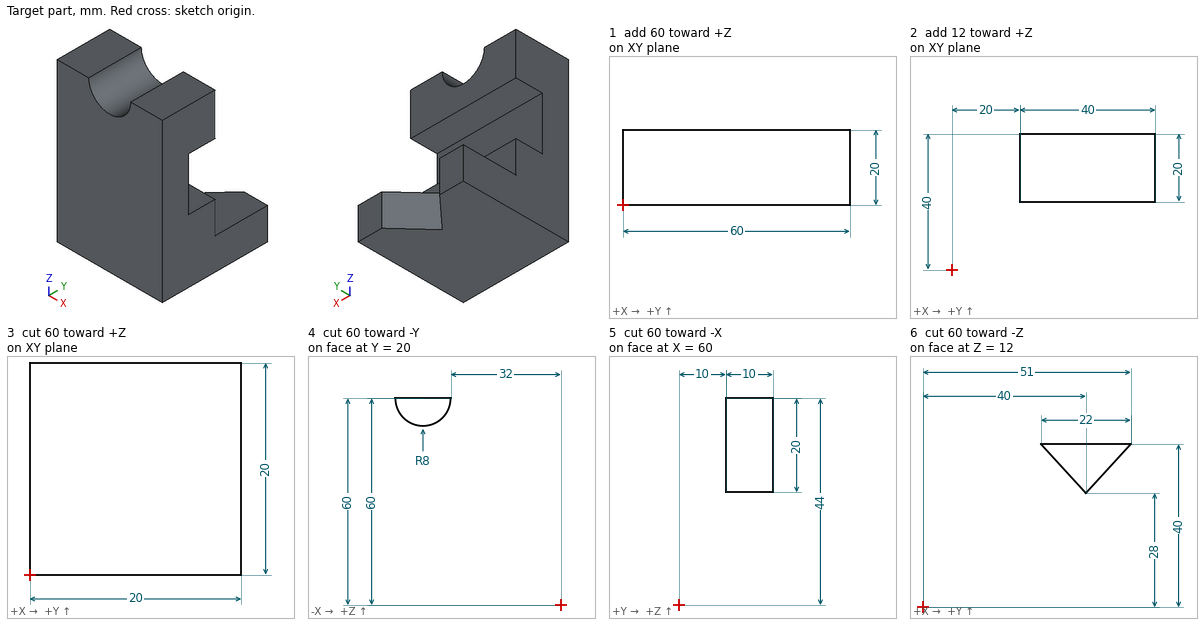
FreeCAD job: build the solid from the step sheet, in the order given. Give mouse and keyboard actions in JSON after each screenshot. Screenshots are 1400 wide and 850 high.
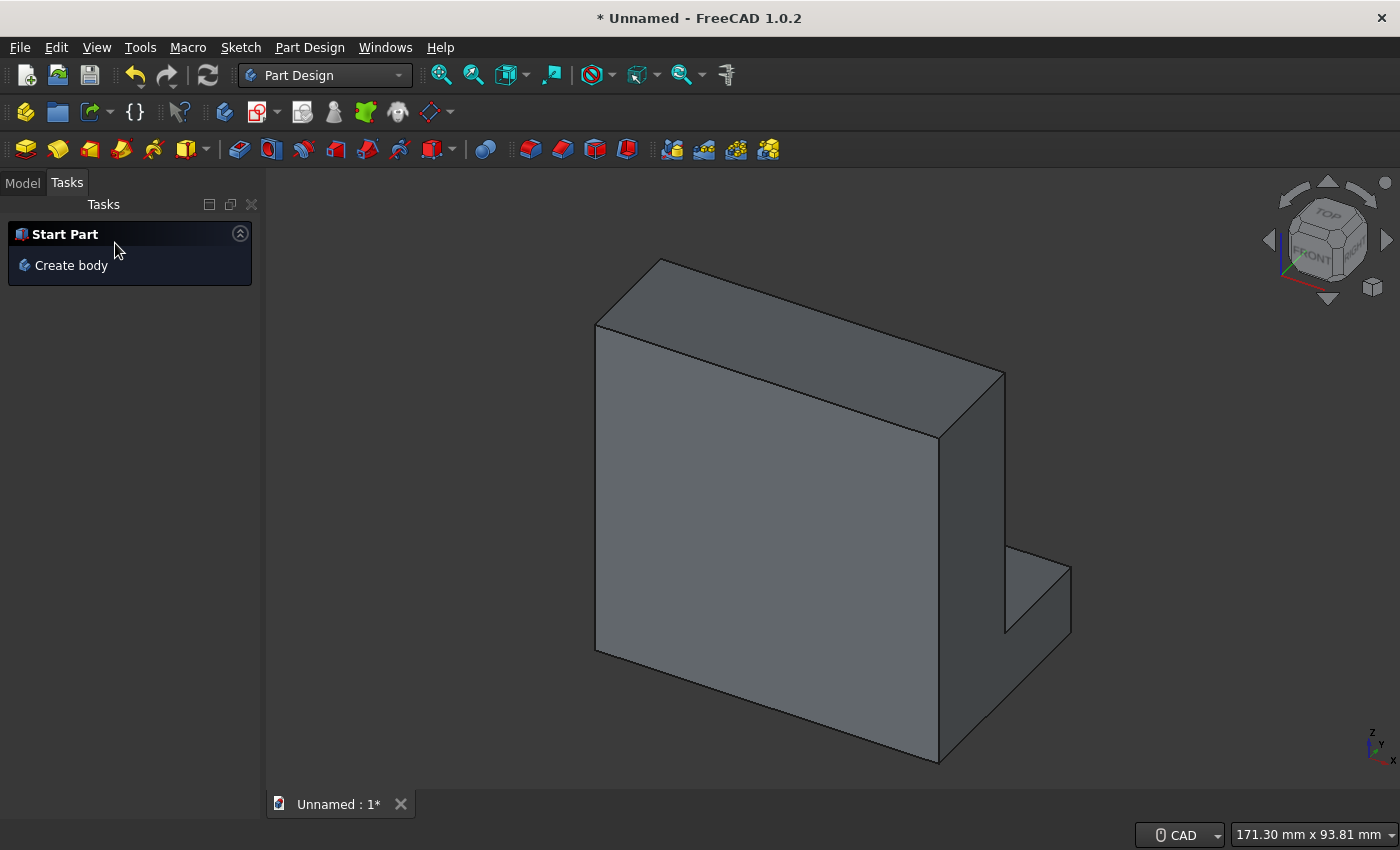
{"action": "left_click", "coordinate": [258, 112]}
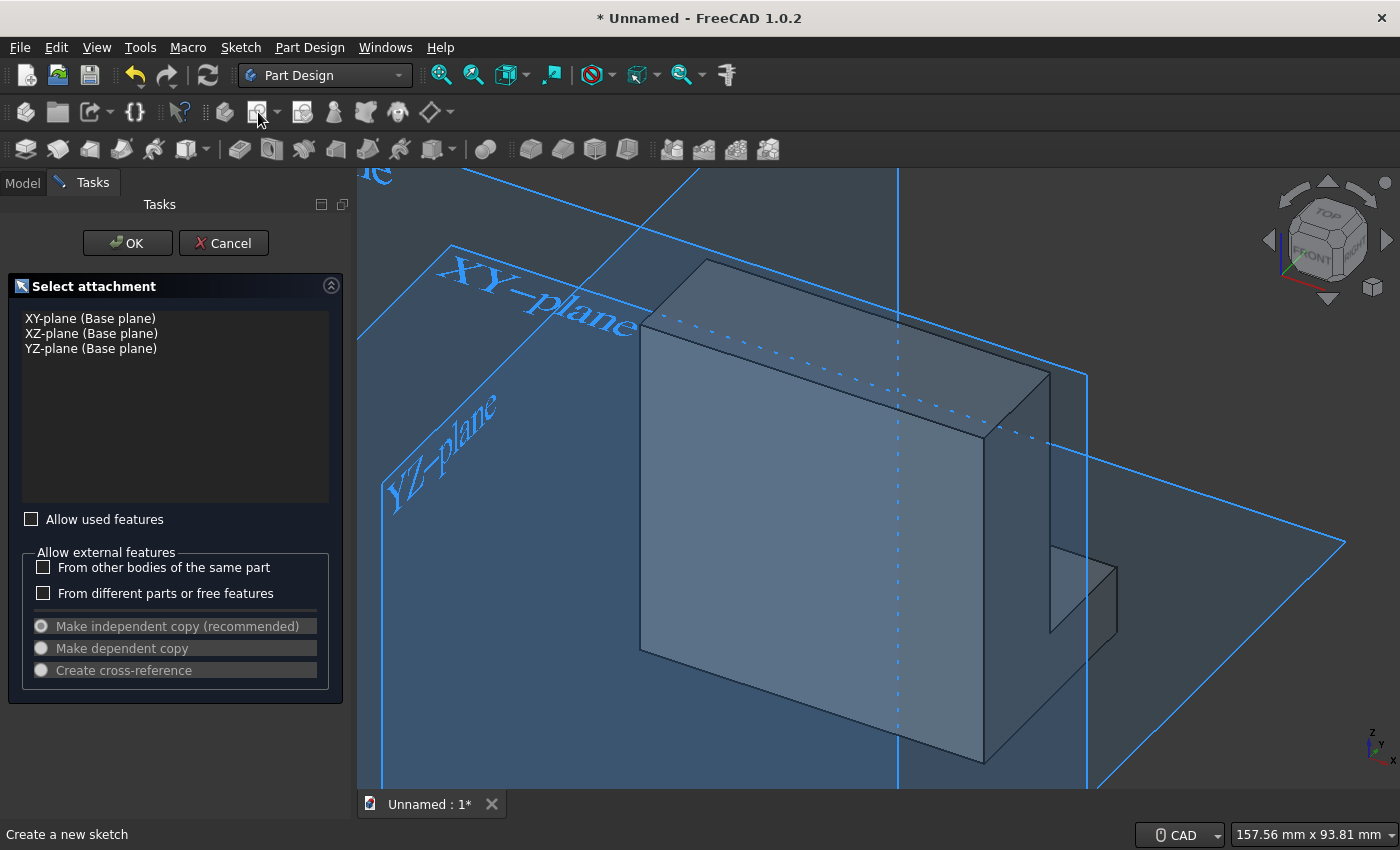
{"action": "left_click", "coordinate": [82, 318]}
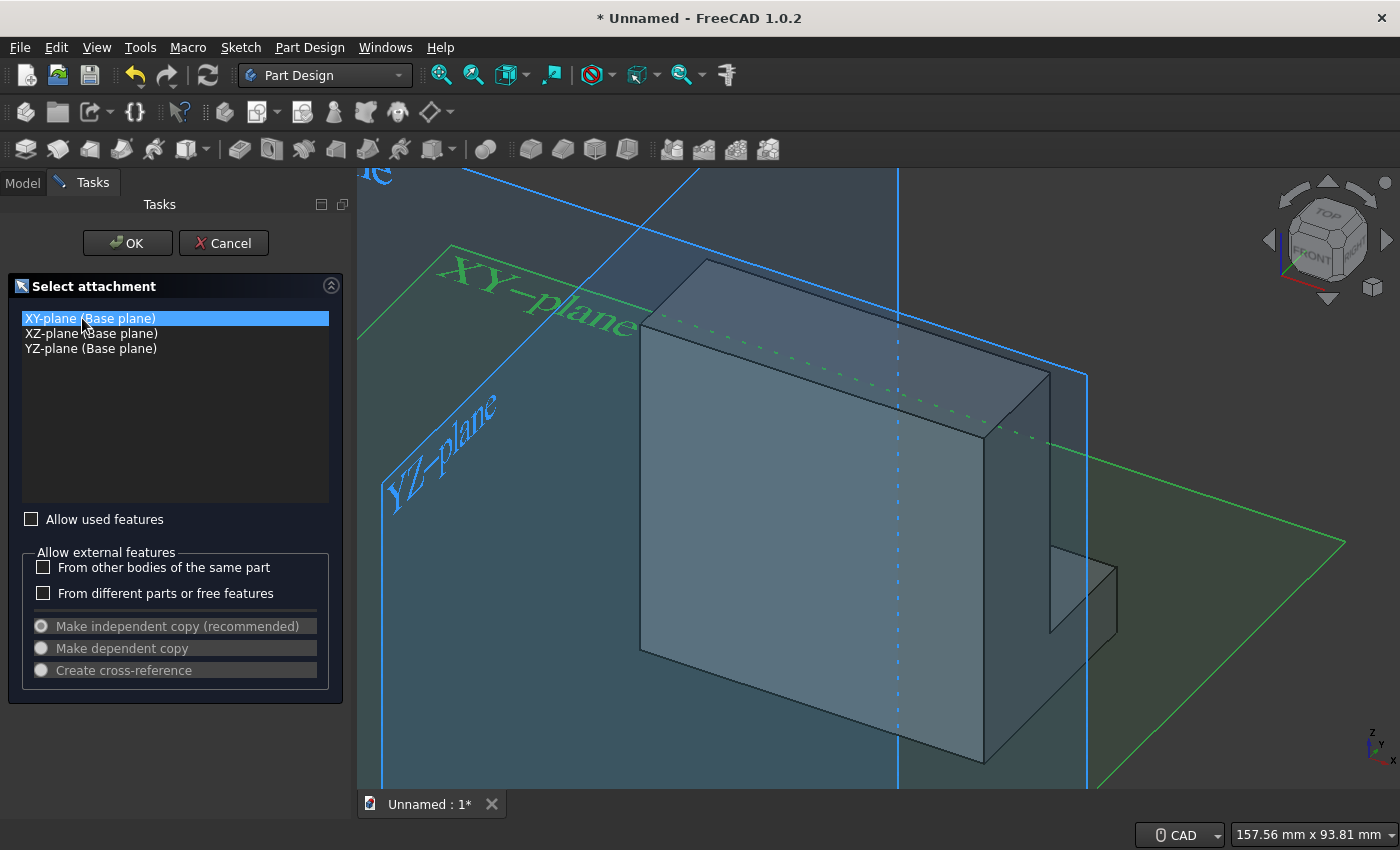
{"action": "left_click", "coordinate": [128, 243]}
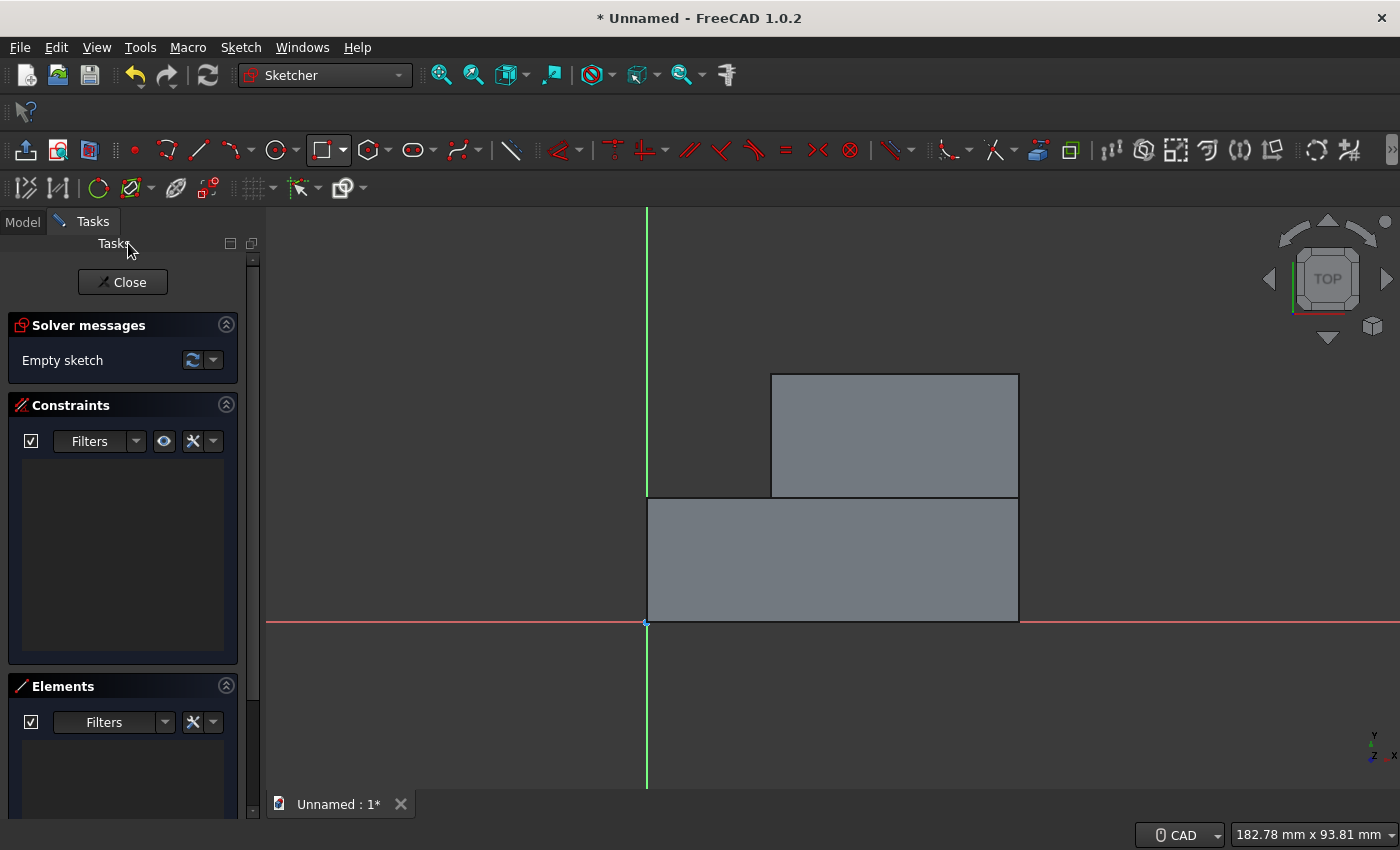
{"action": "left_click", "coordinate": [90, 150]}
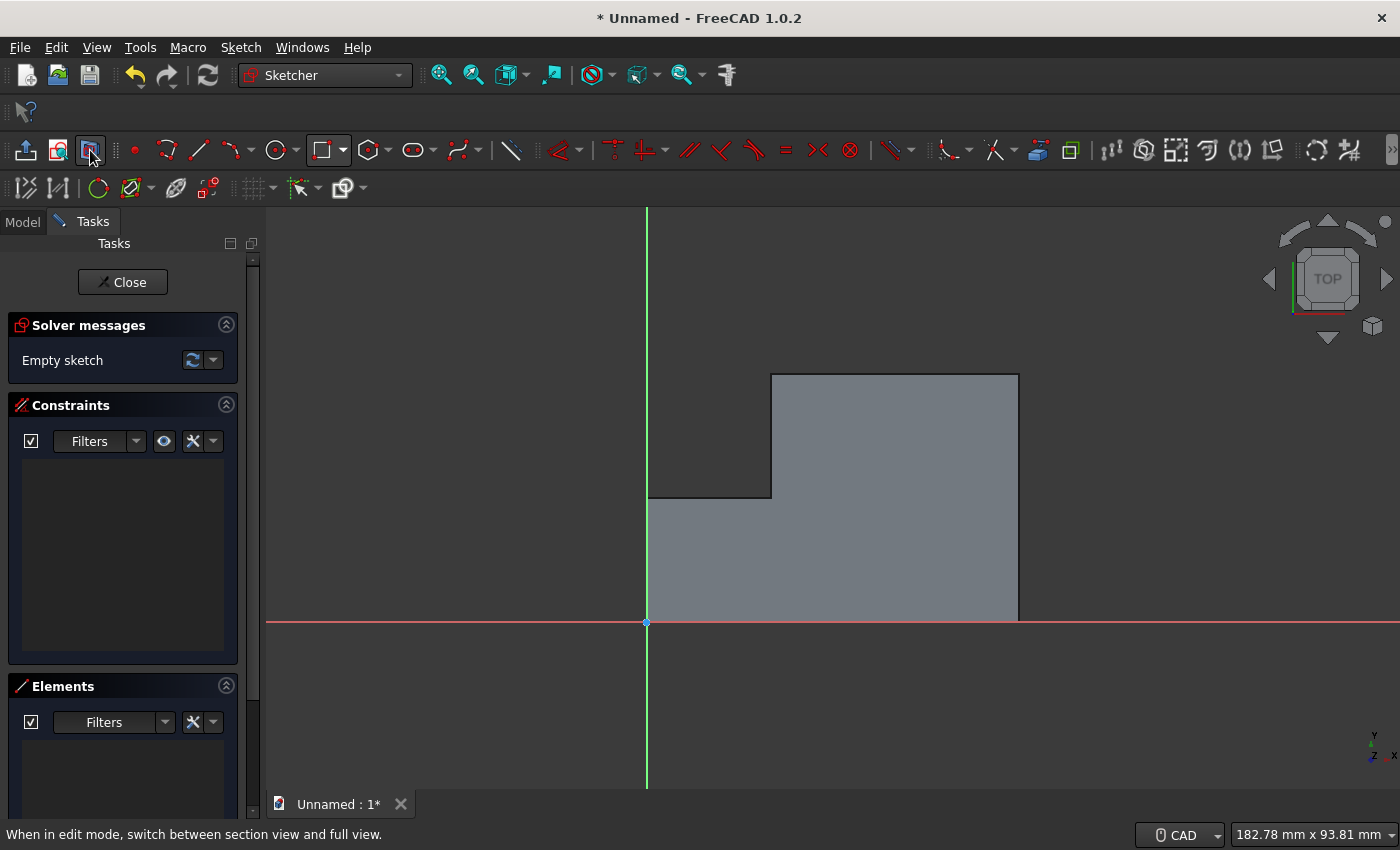
{"action": "scroll", "coordinate": [677, 596], "scroll_direction": "up", "scroll_amount": 5}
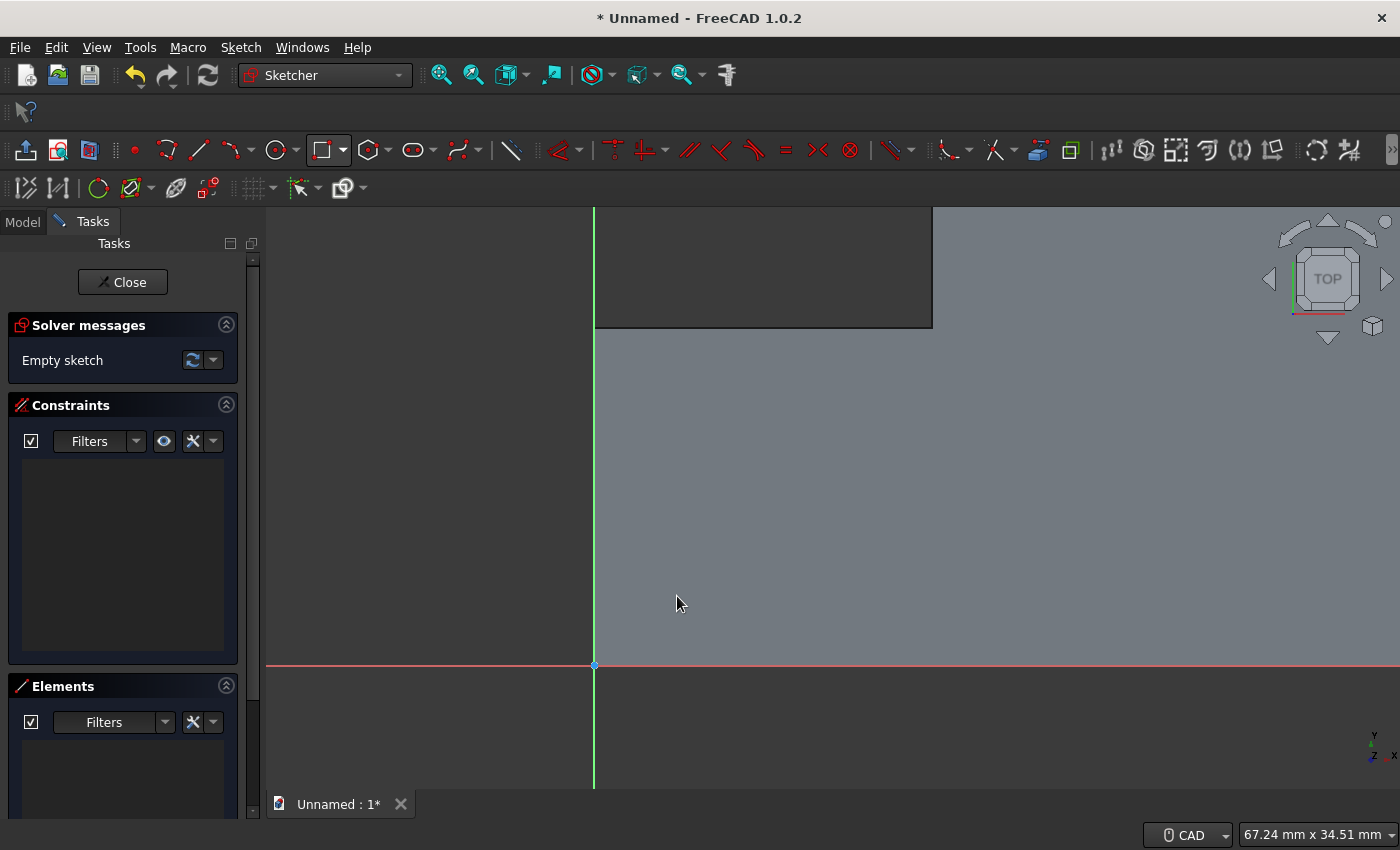
{"action": "left_click", "coordinate": [322, 150]}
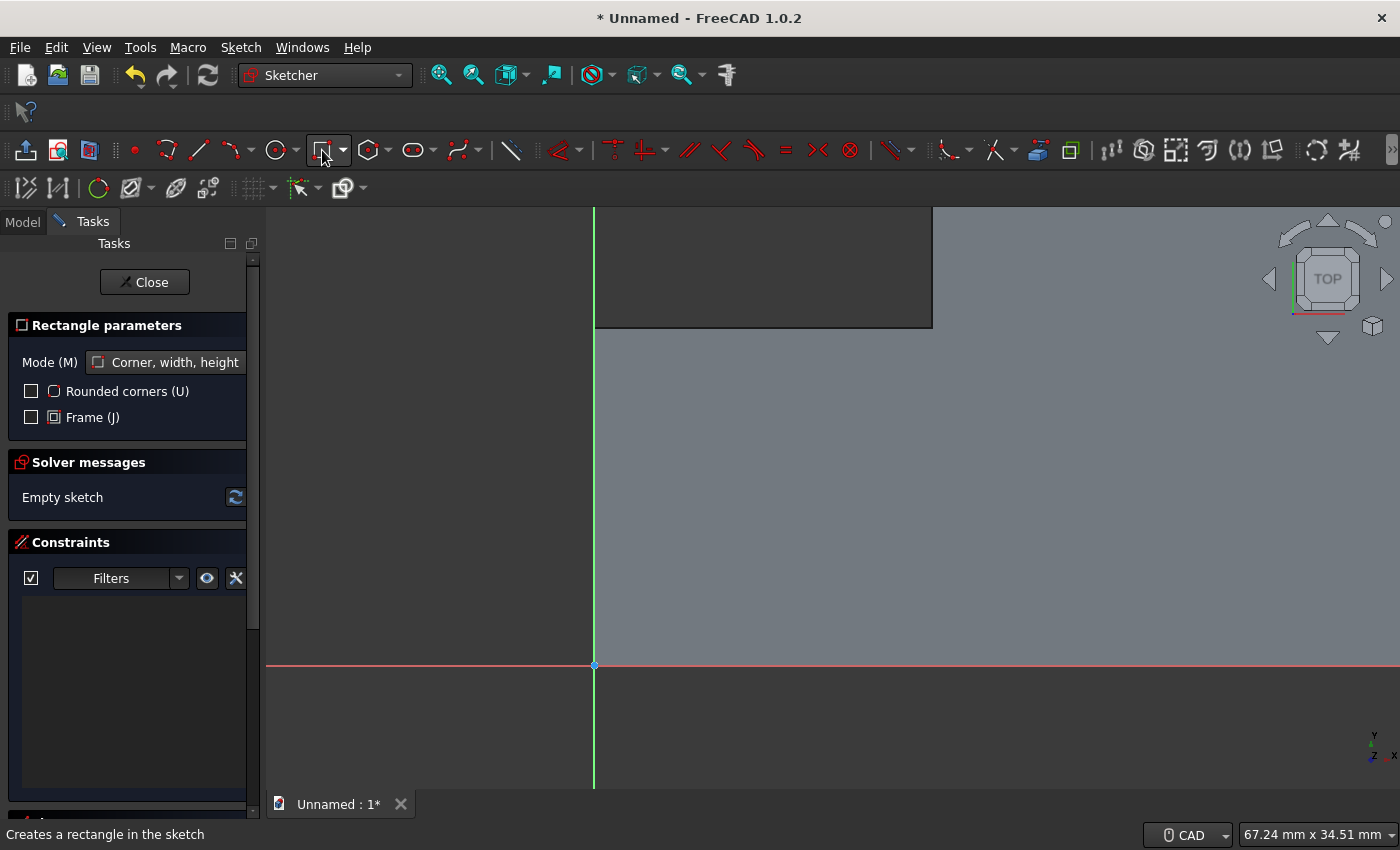
{"action": "left_click", "coordinate": [594, 666]}
{"action": "mouse_move", "coordinate": [932, 328]}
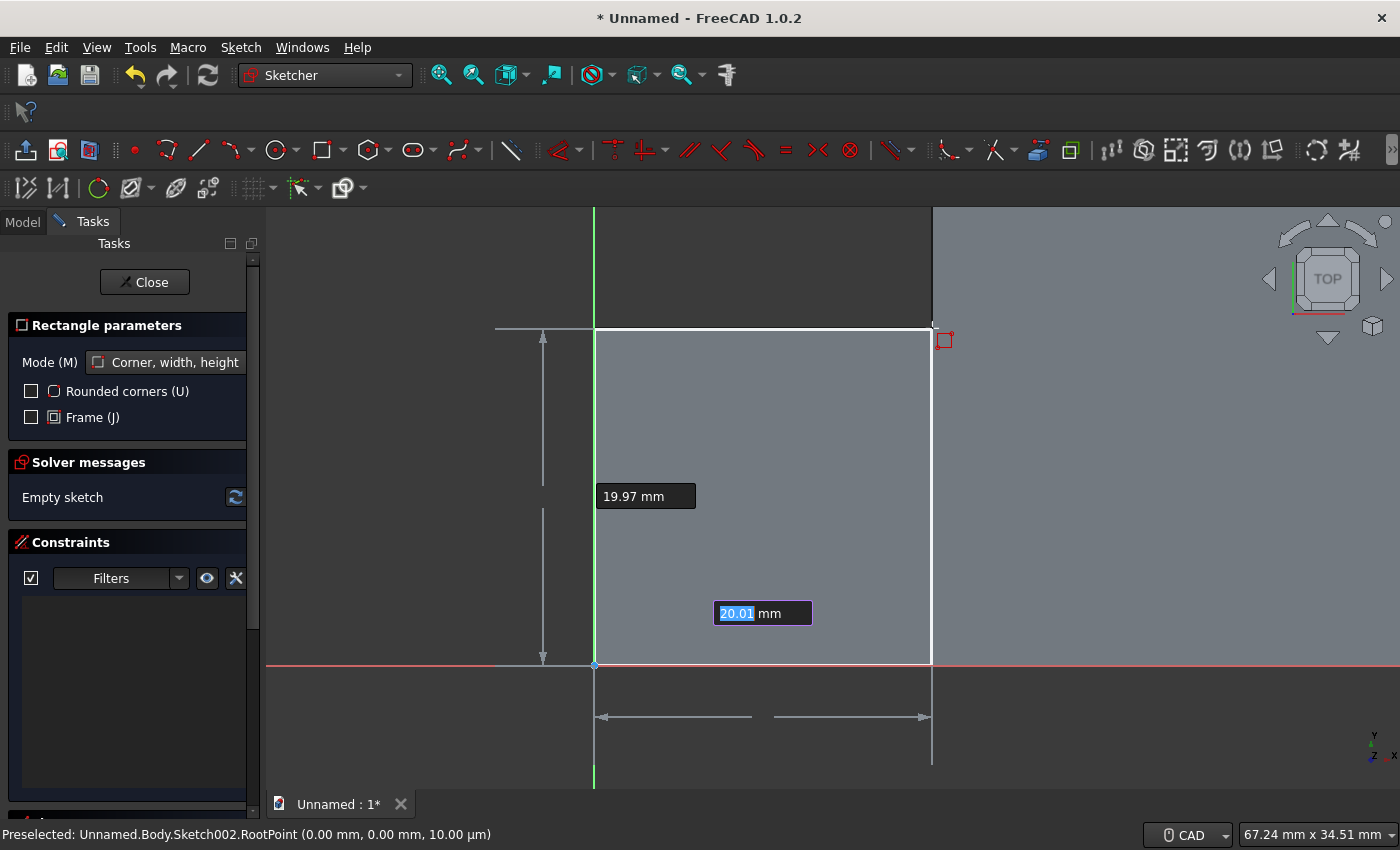
{"action": "type", "text": "20"}
{"action": "key", "text": "Tab"}
{"action": "type", "text": "20"}
{"action": "key", "text": "Return"}
{"action": "key", "text": "Escape"}